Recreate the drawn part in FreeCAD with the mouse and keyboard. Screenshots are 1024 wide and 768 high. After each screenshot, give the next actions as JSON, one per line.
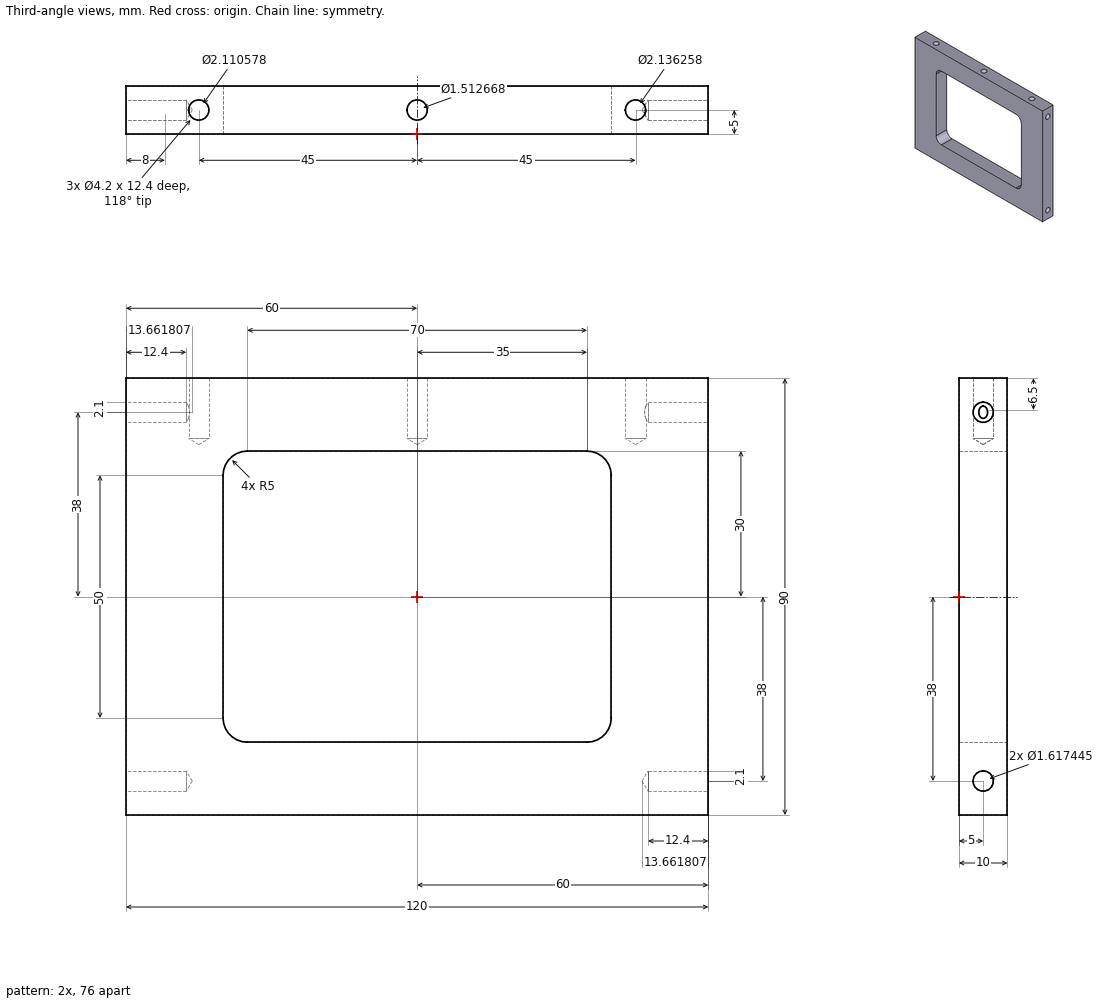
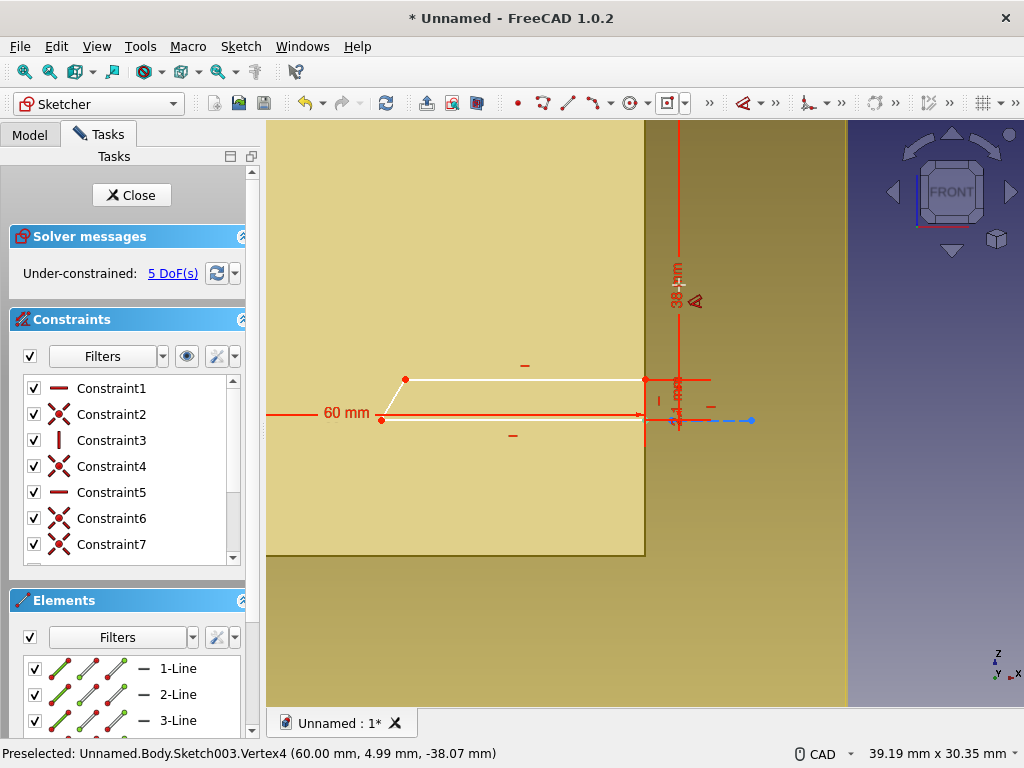
{"action": "left_click", "coordinate": [671, 421]}
{"action": "left_click", "coordinate": [705, 222]}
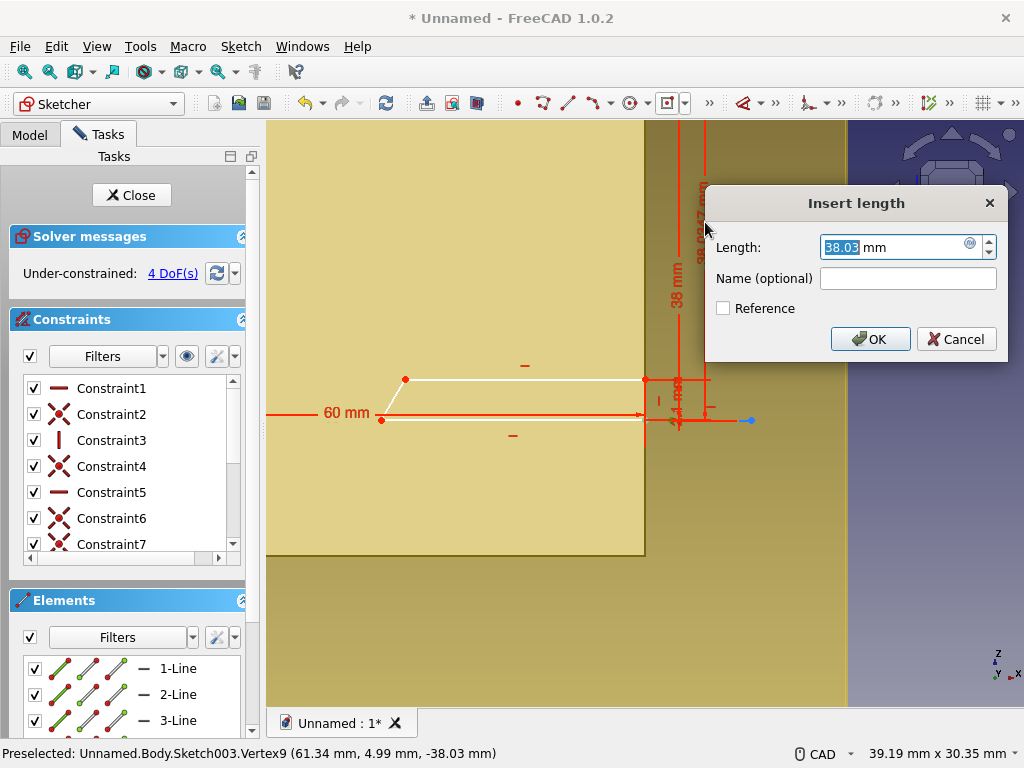
{"action": "type", "text": "38"}
{"action": "key", "text": "Return"}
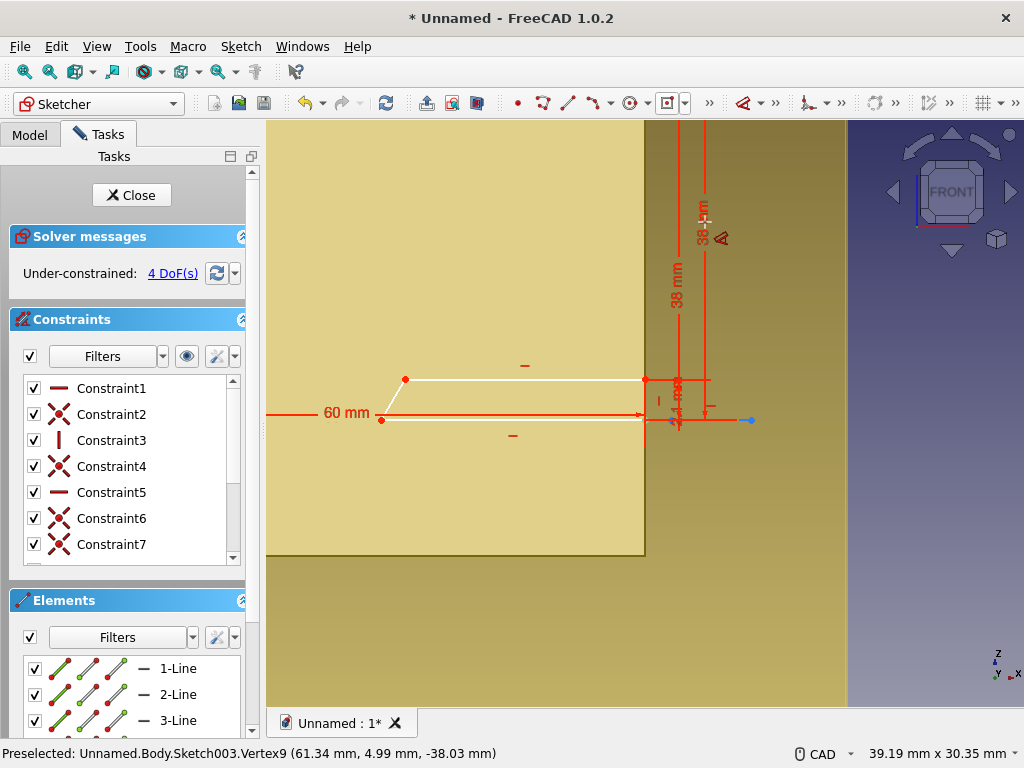
{"action": "left_click", "coordinate": [477, 380]}
{"action": "left_click", "coordinate": [525, 346]}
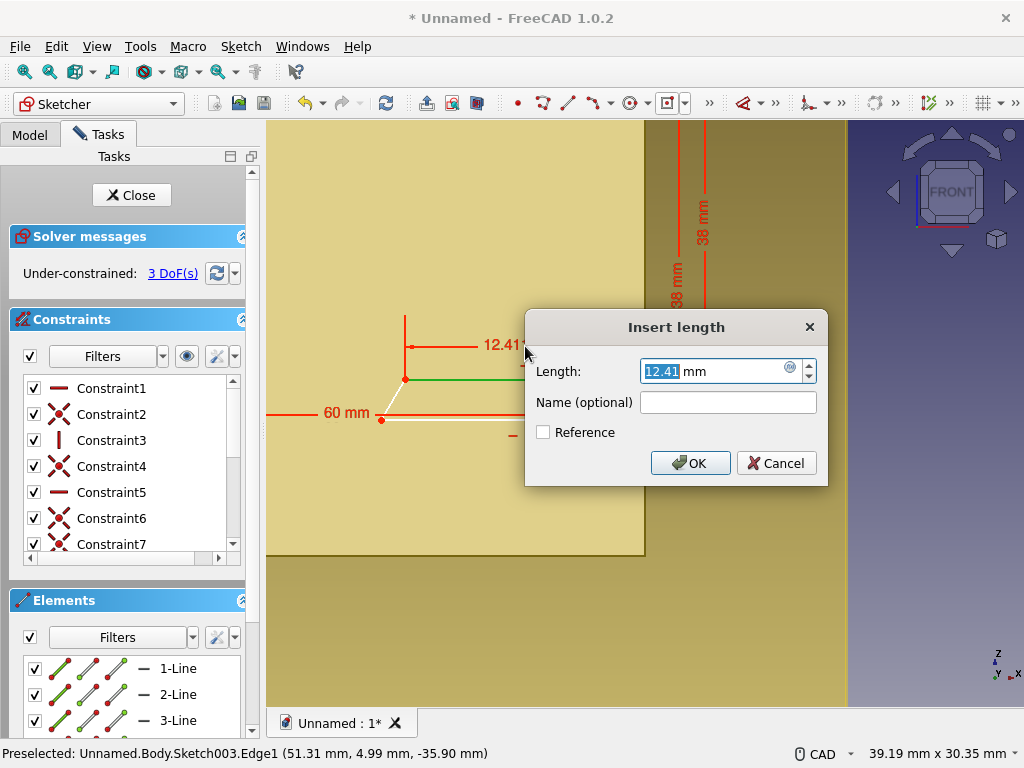
{"action": "type", "text": "12.4"}
{"action": "key", "text": "Return"}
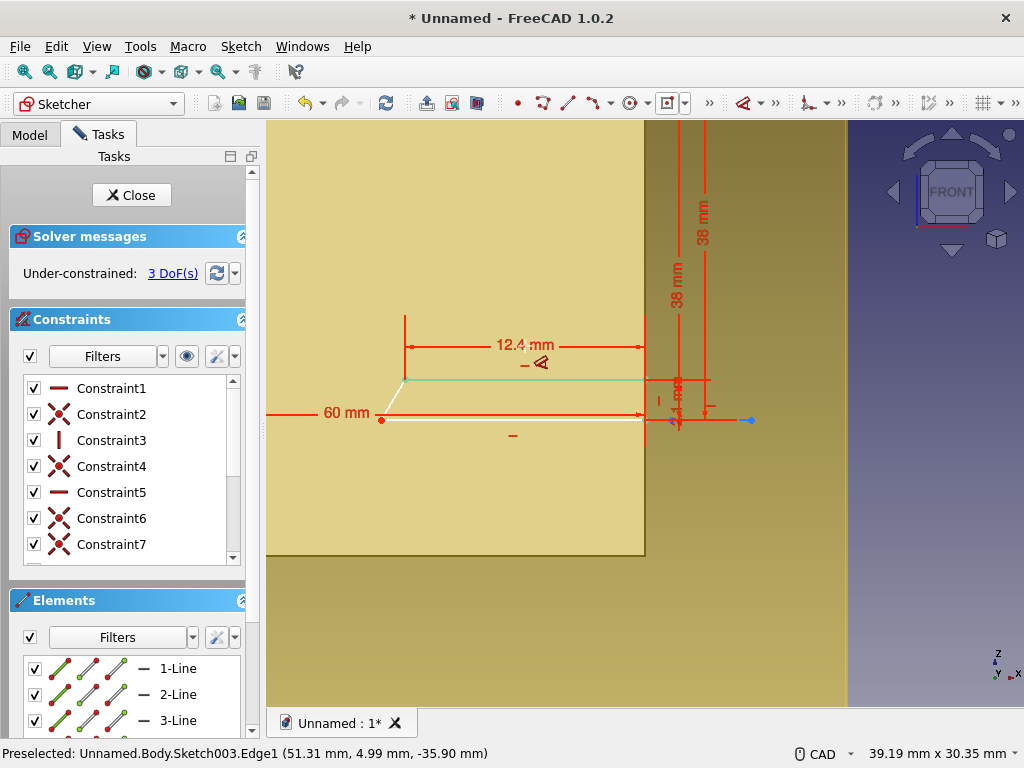
{"action": "left_click", "coordinate": [566, 420]}
{"action": "left_click", "coordinate": [513, 454]}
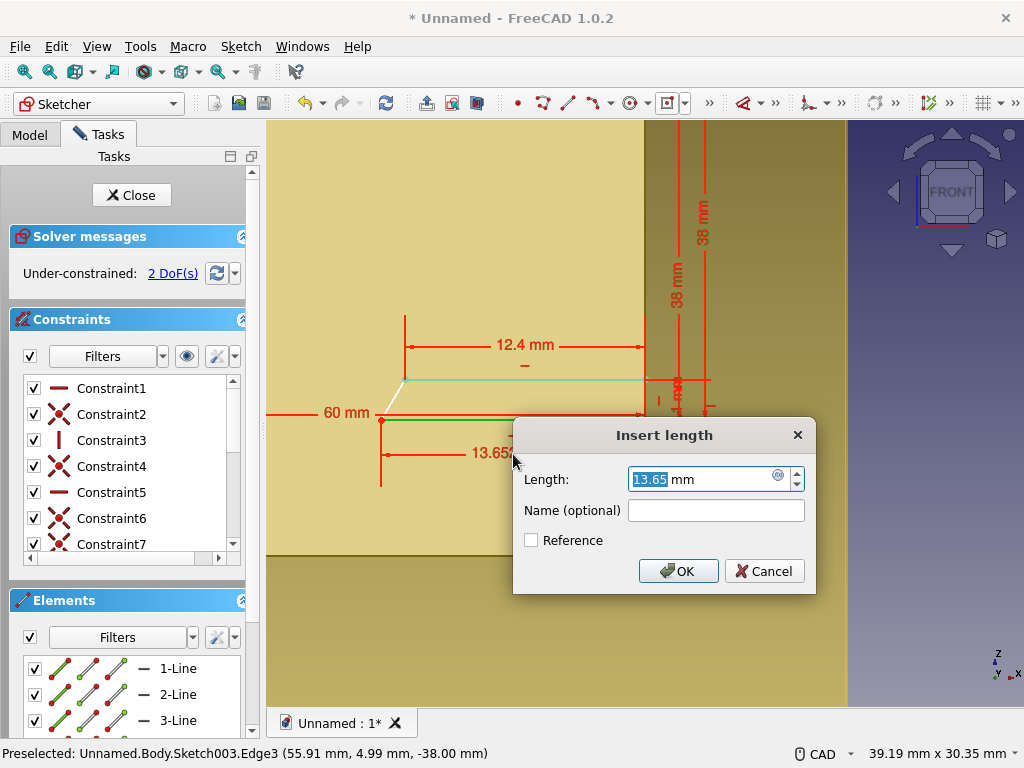
{"action": "type", "text": "13.661807"}
{"action": "key", "text": "Return"}
{"action": "key", "text": "Escape"}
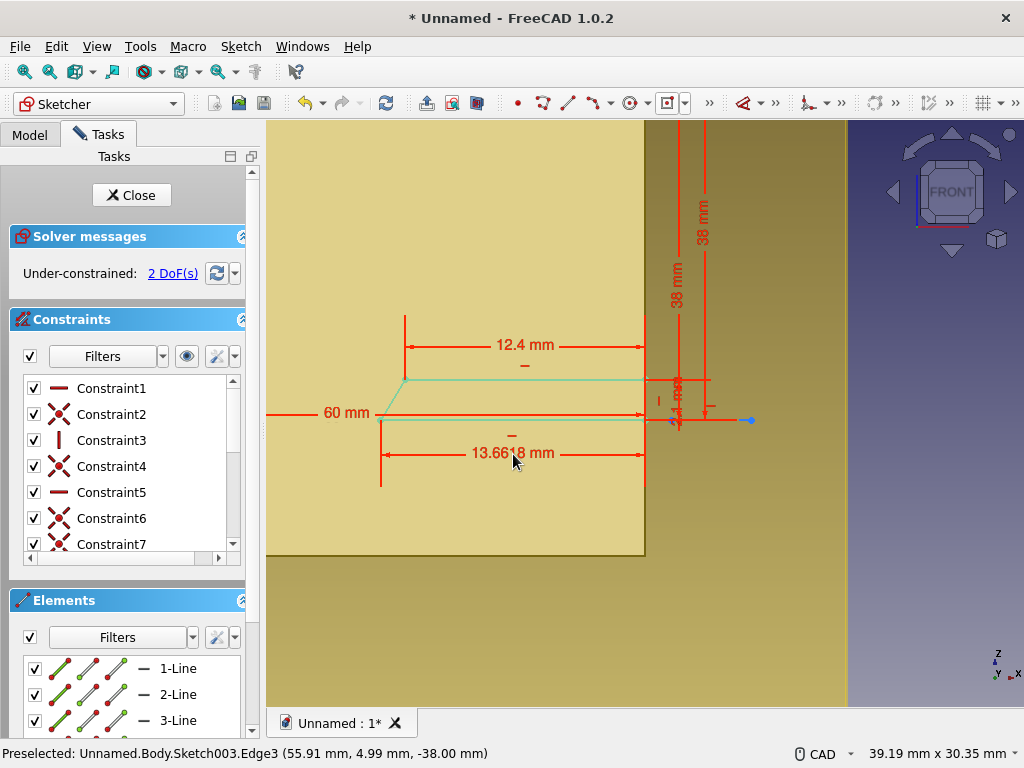
{"action": "left_click", "coordinate": [132, 195]}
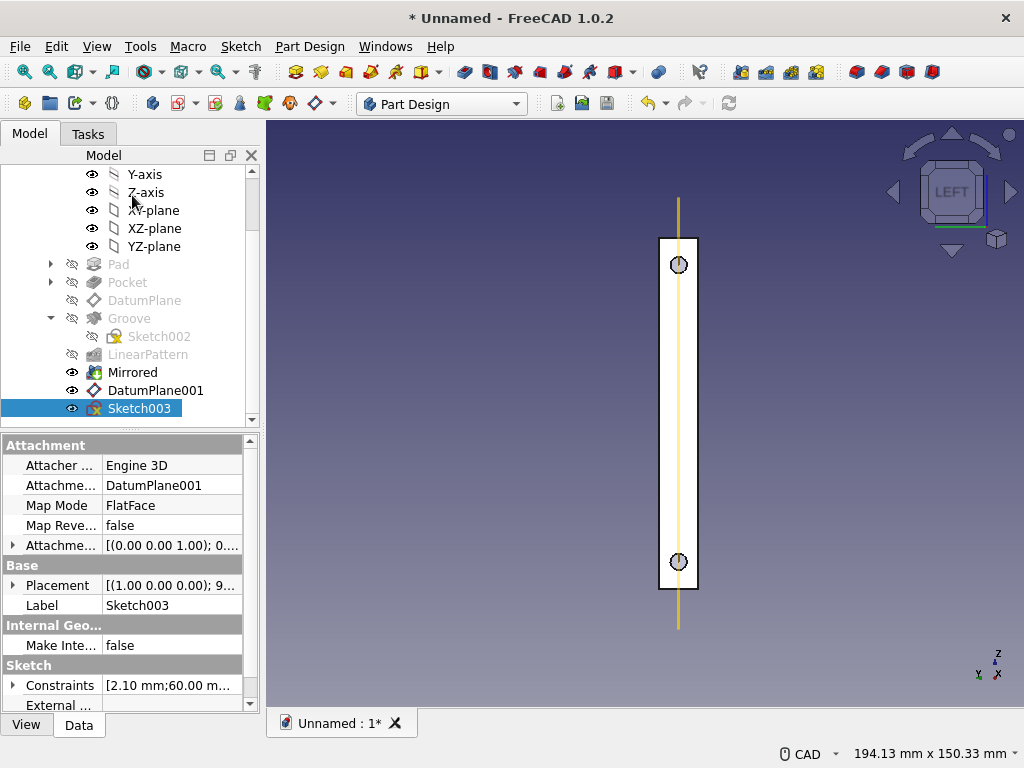
{"action": "left_click", "coordinate": [515, 72]}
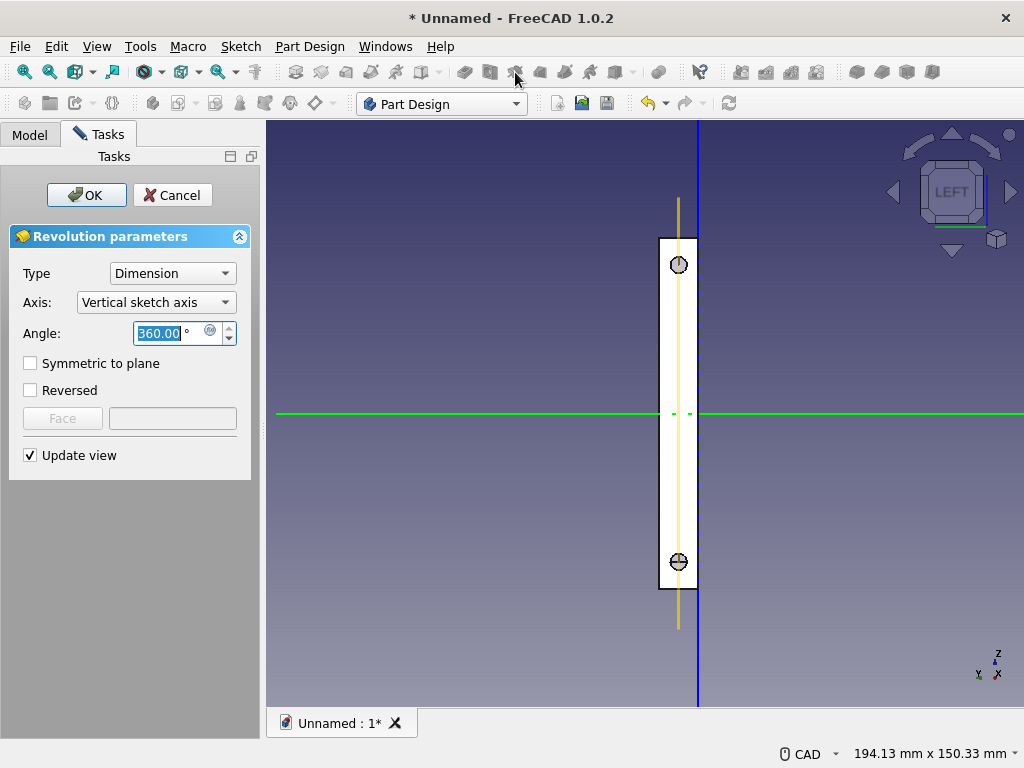
{"action": "left_click", "coordinate": [157, 302]}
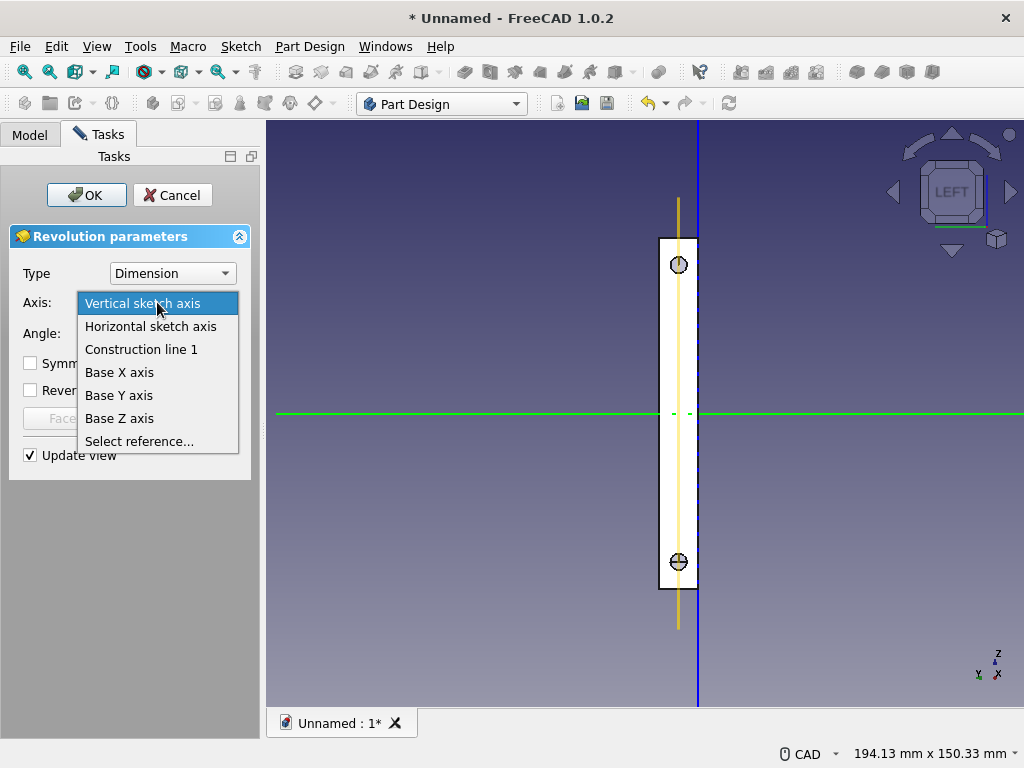
{"action": "left_click", "coordinate": [156, 350]}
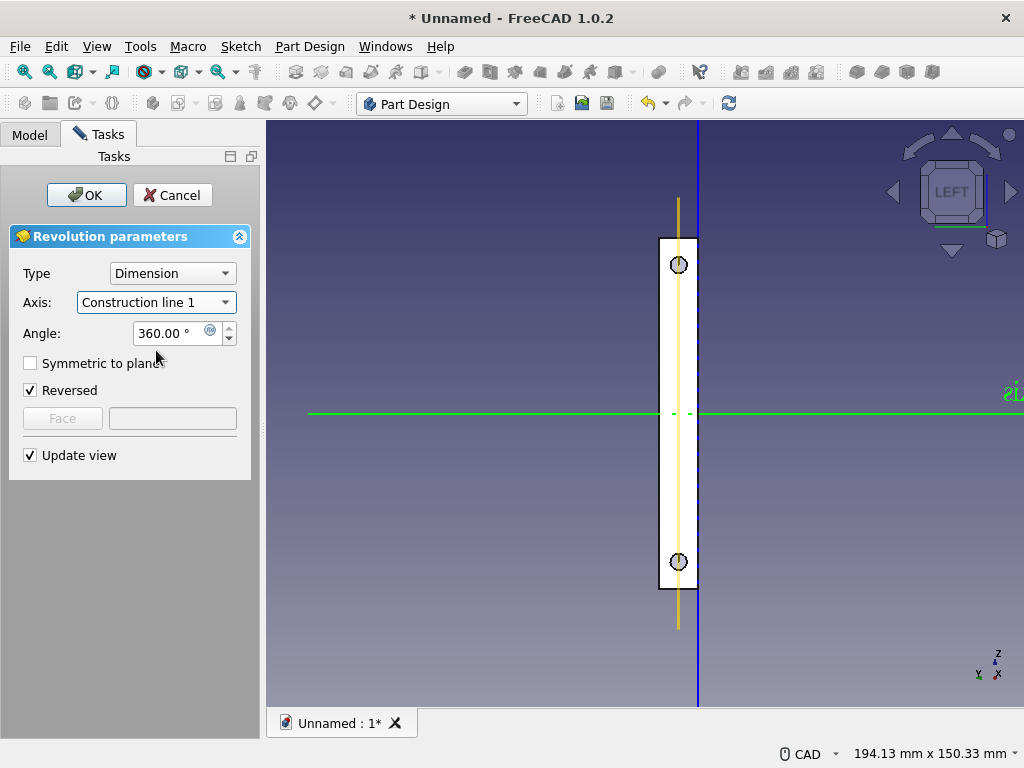
{"action": "left_click", "coordinate": [87, 195]}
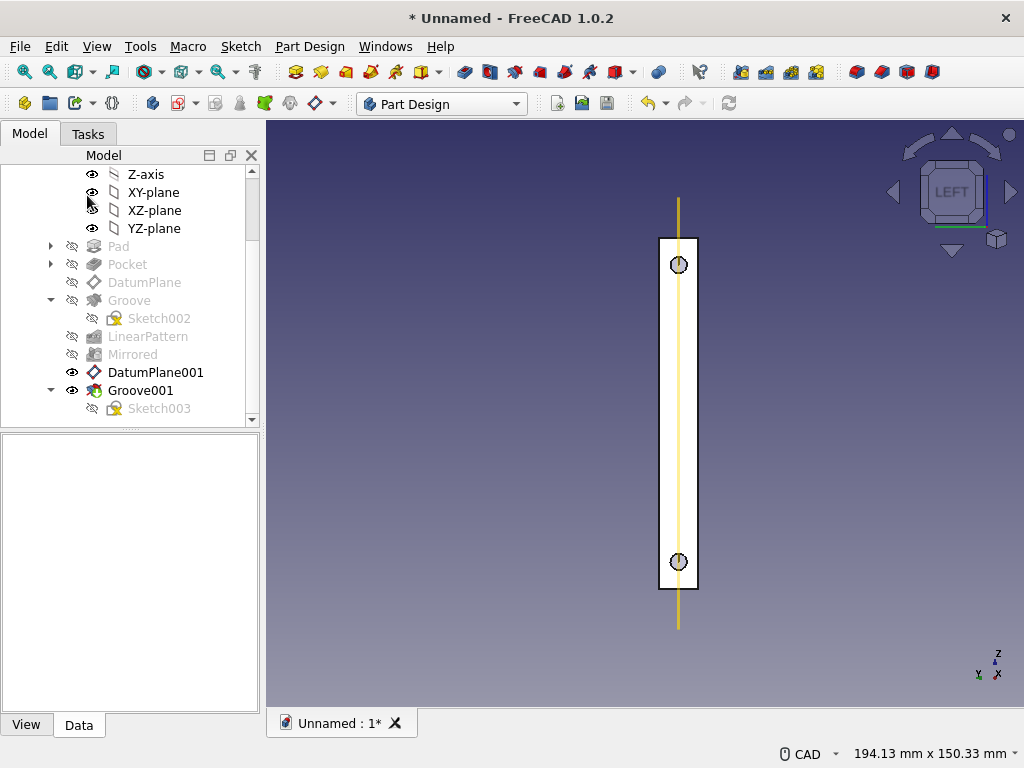
{"action": "left_click", "coordinate": [117, 372]}
{"action": "key", "text": "space"}